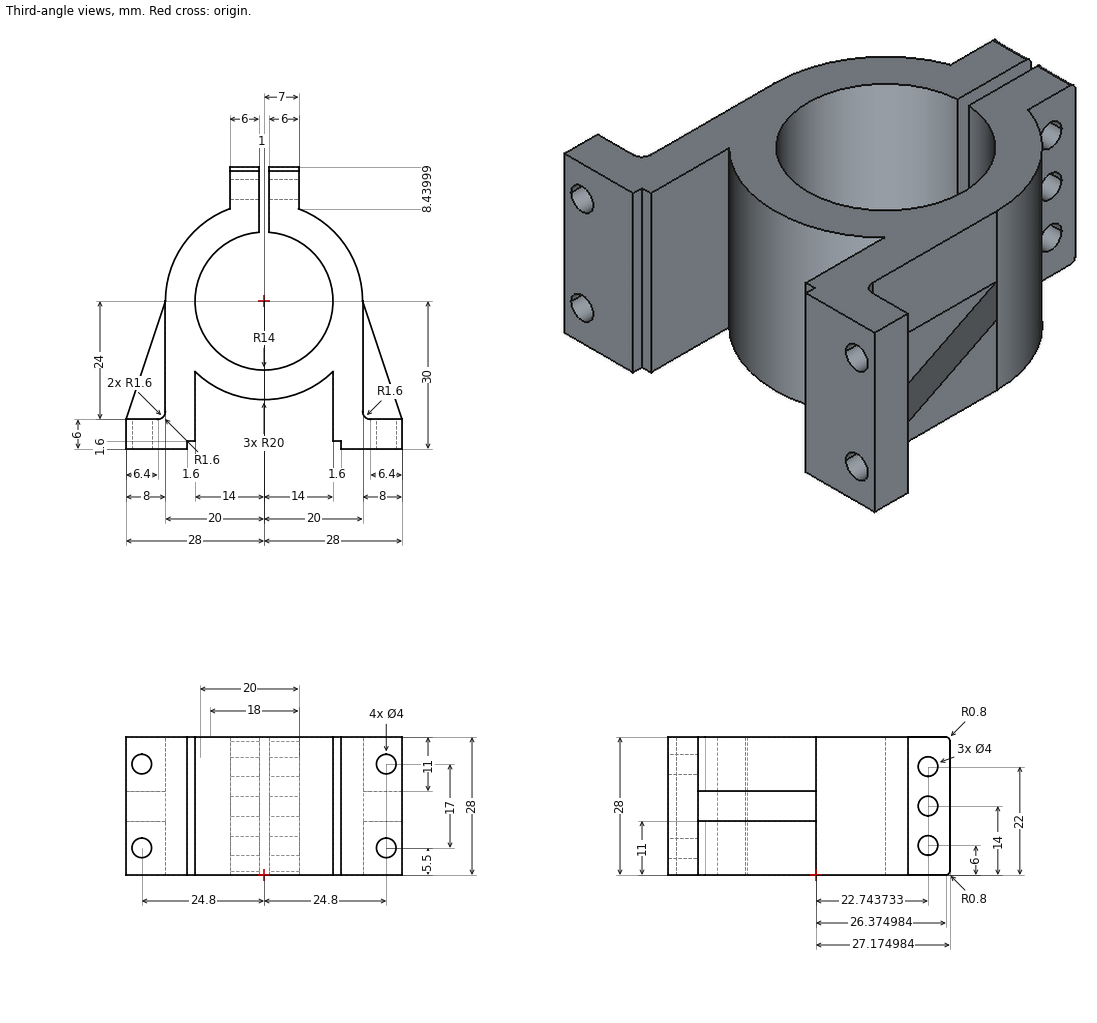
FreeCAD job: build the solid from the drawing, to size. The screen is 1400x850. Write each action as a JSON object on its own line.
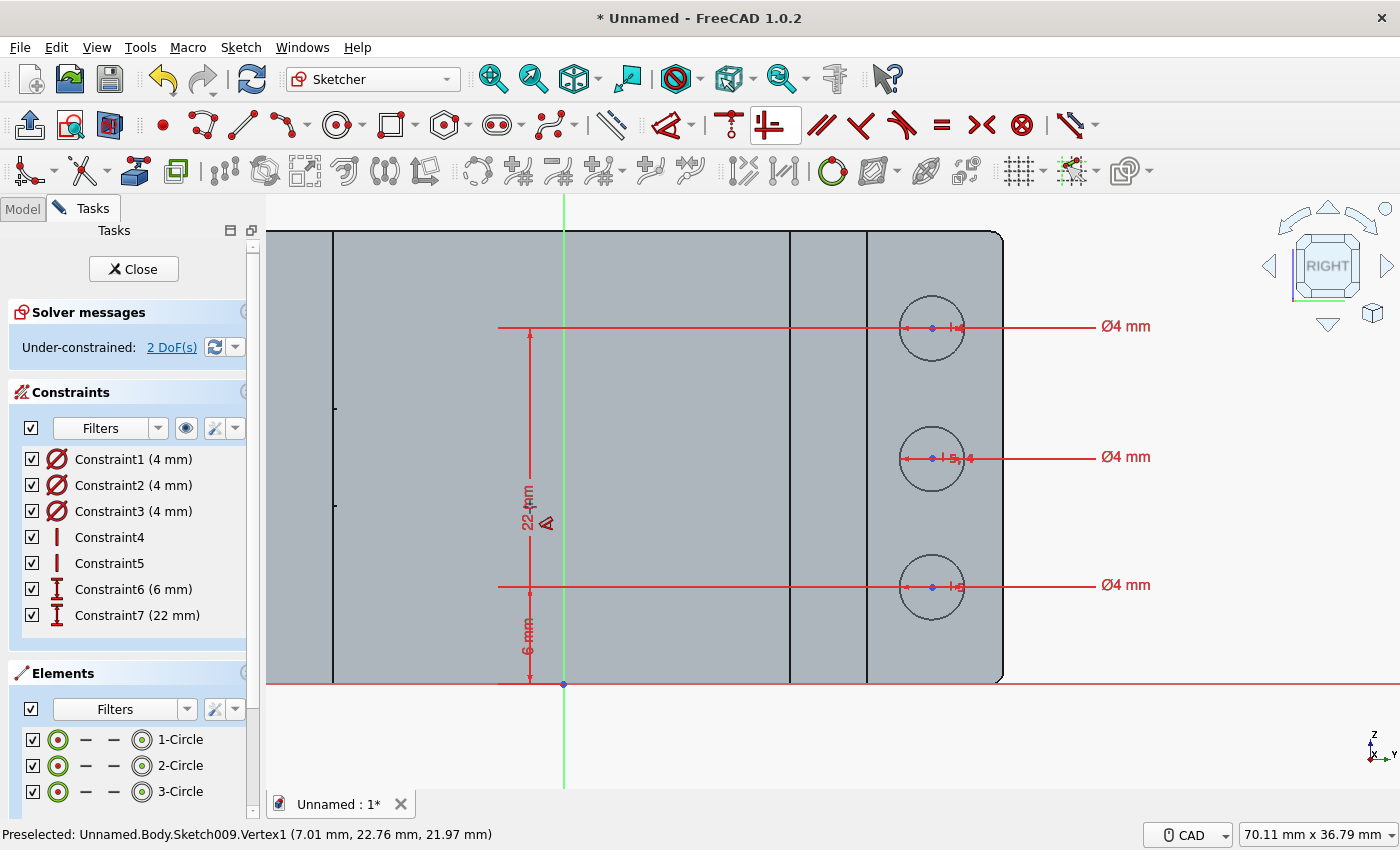
{"action": "left_click", "coordinate": [932, 459]}
{"action": "left_click", "coordinate": [530, 572]}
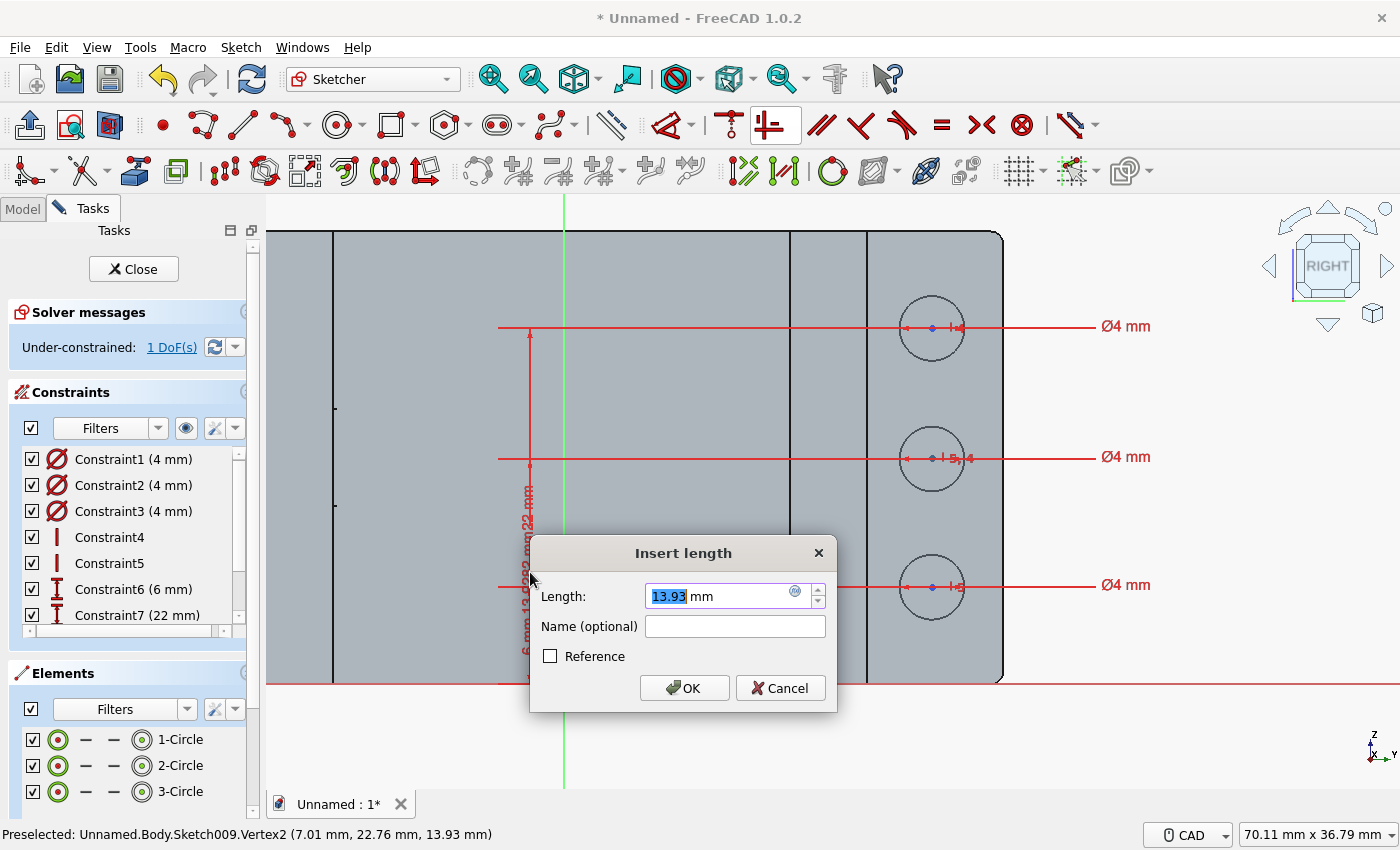
{"action": "type", "text": "14"}
{"action": "key", "text": "Return"}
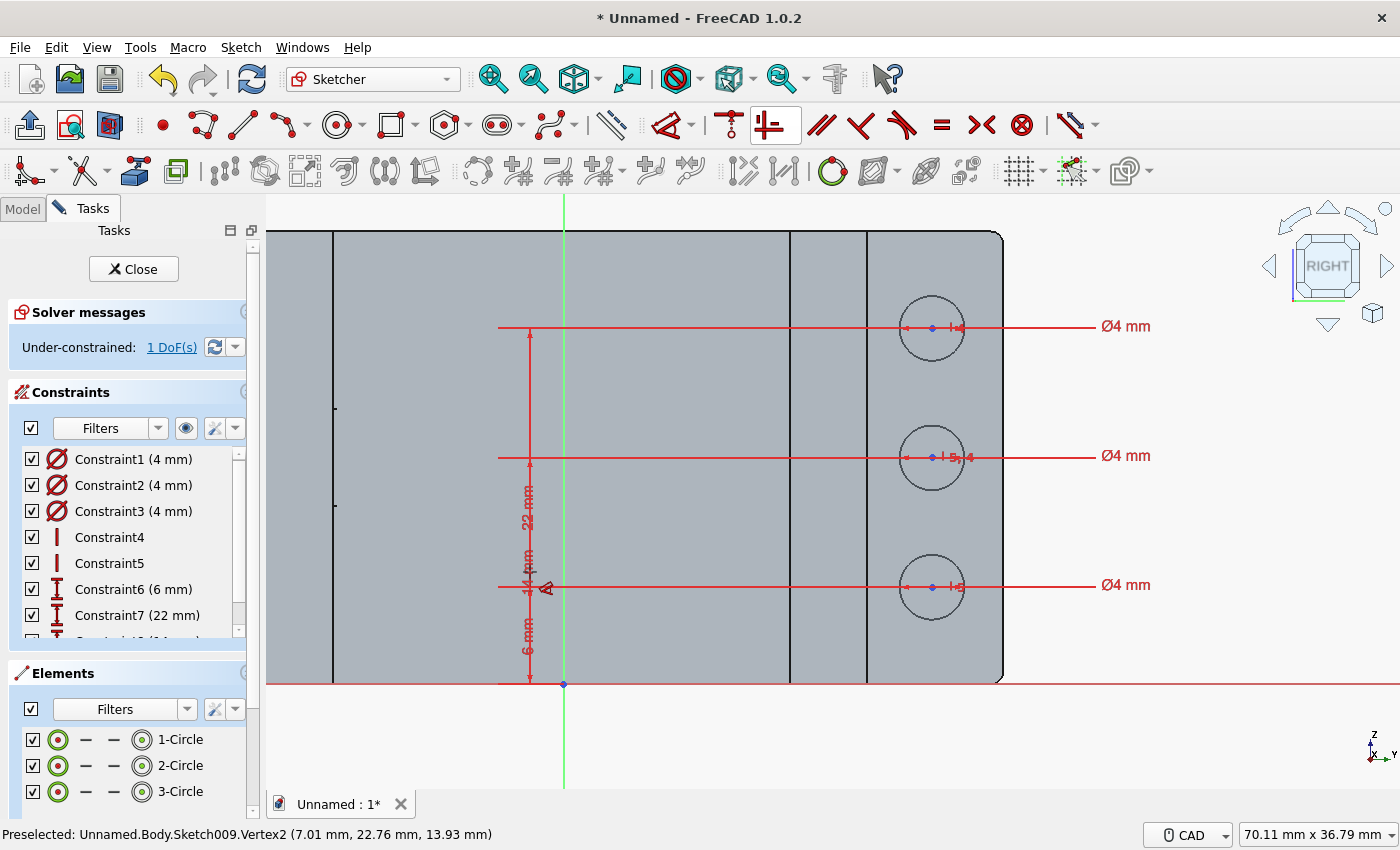
{"action": "left_click", "coordinate": [932, 328]}
{"action": "left_click", "coordinate": [748, 718]}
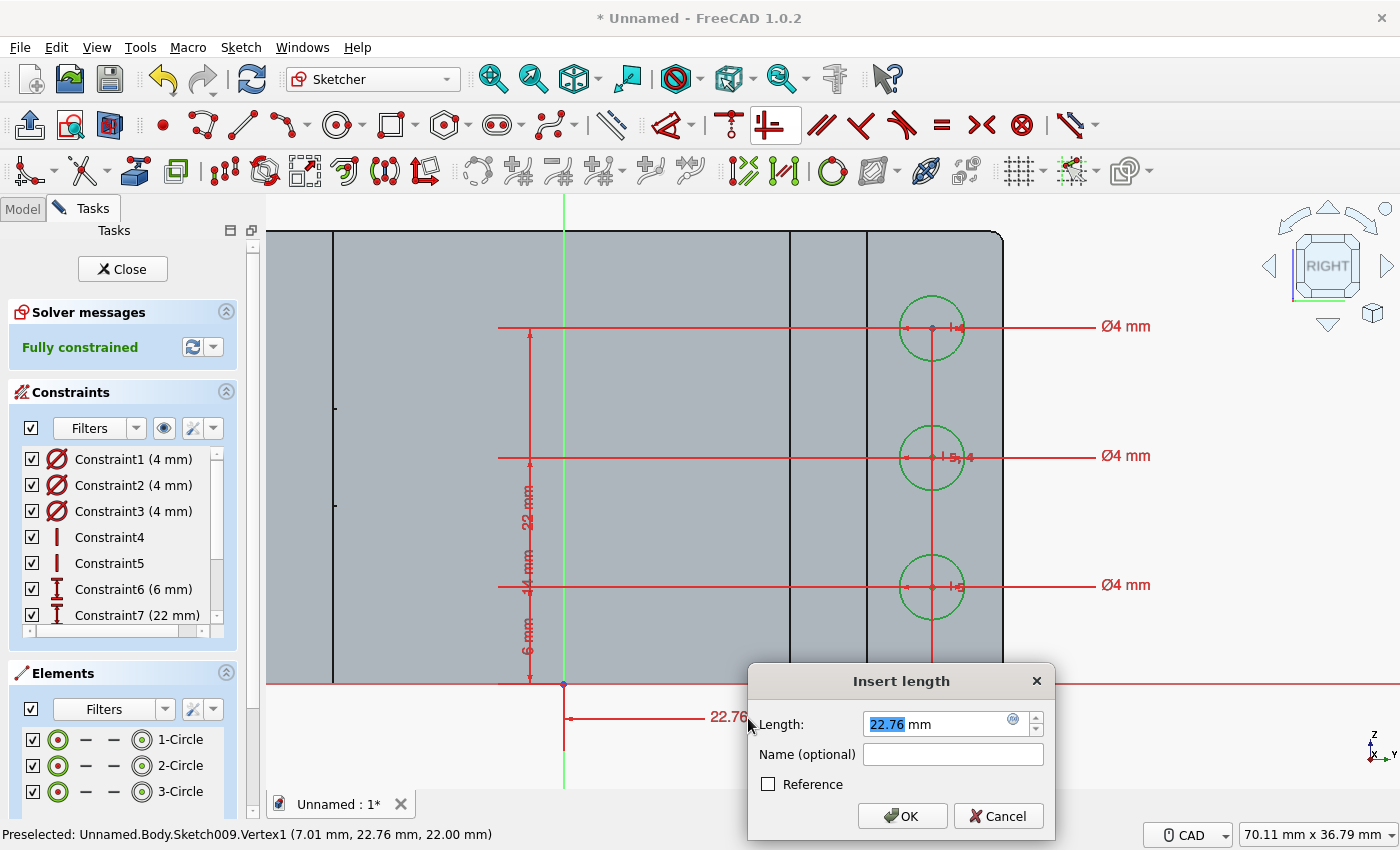
{"action": "type", "text": "22.743733"}
{"action": "key", "text": "Return"}
{"action": "key", "text": "Escape"}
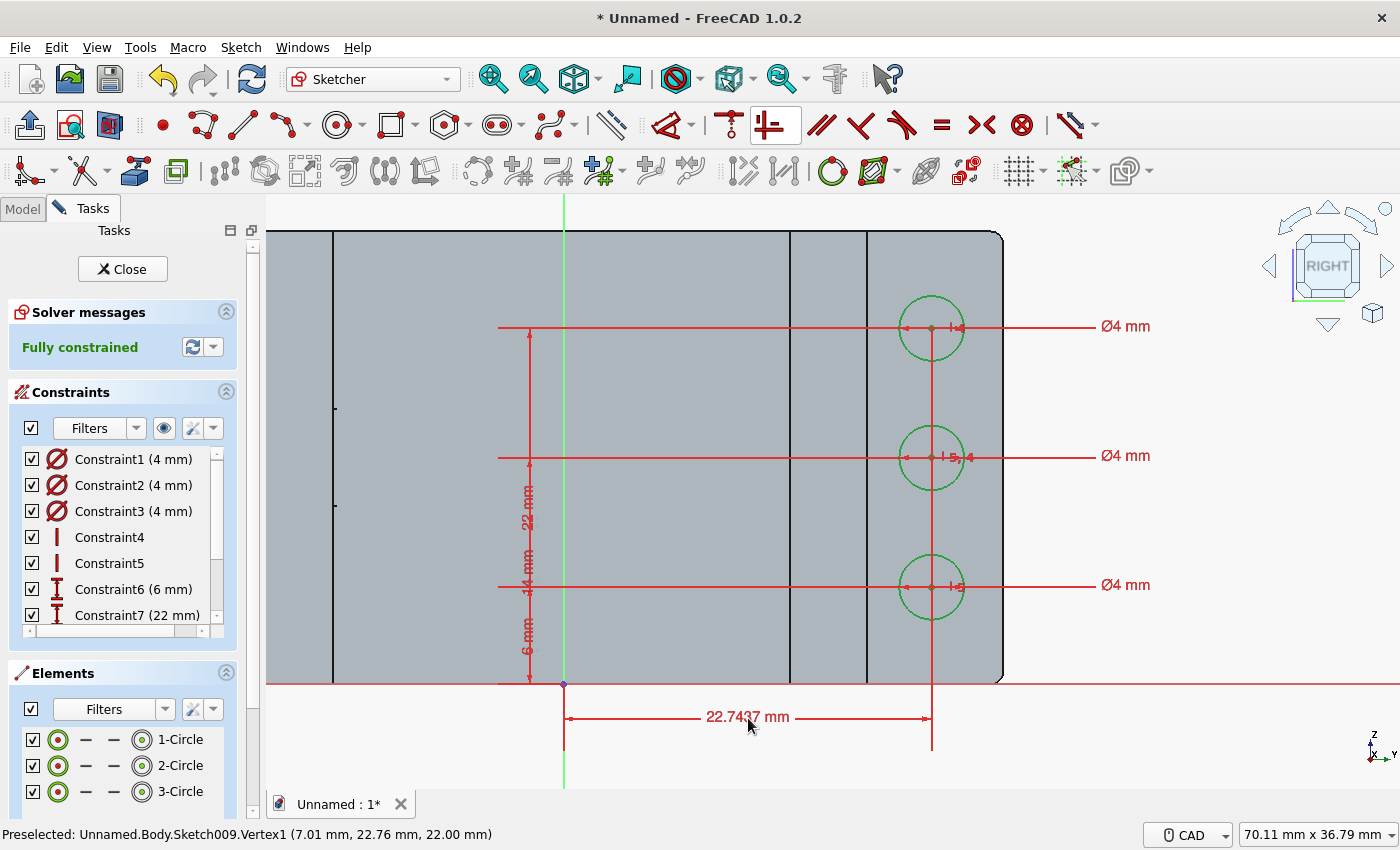
{"action": "left_click", "coordinate": [123, 269]}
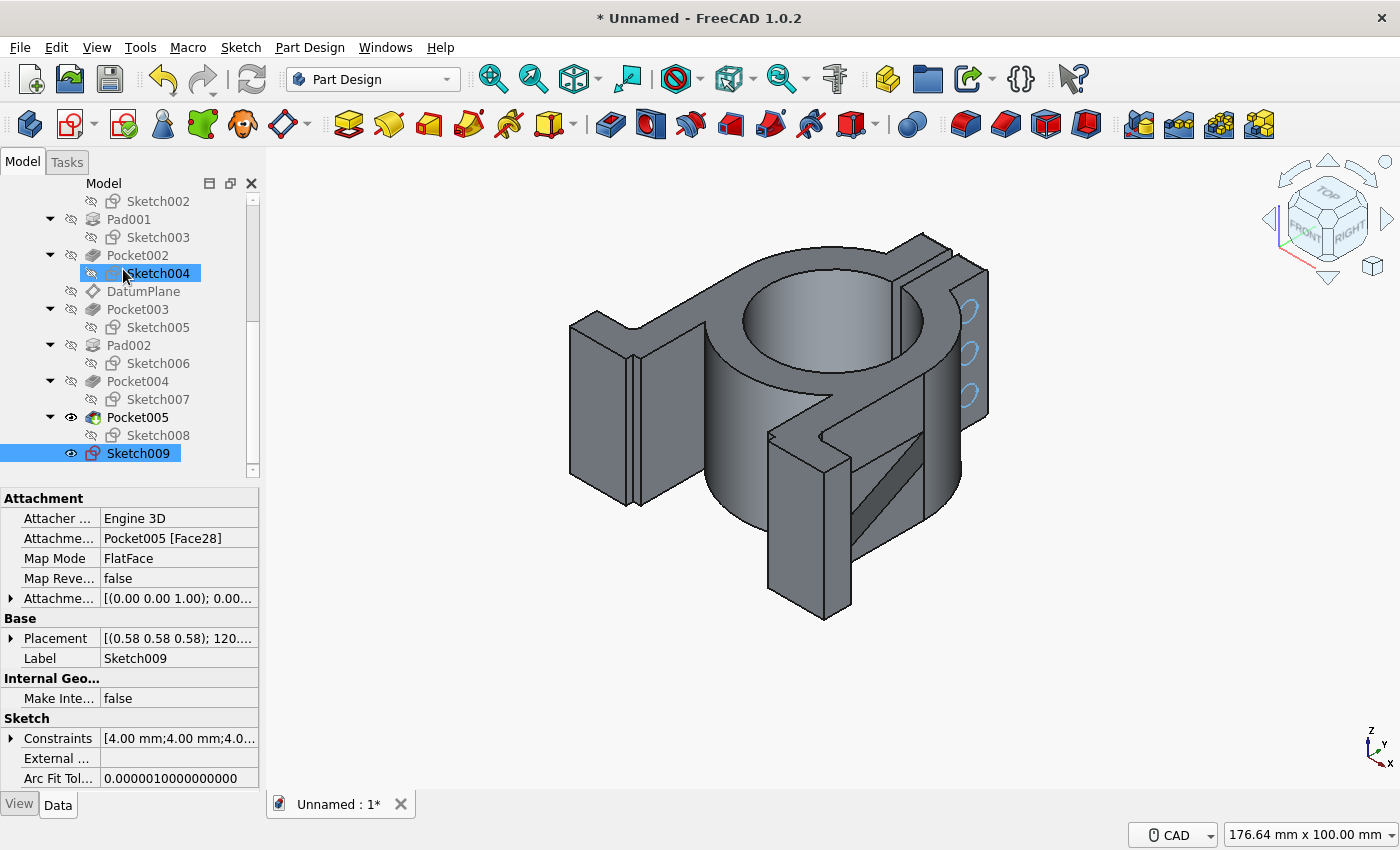
{"action": "left_click", "coordinate": [612, 124]}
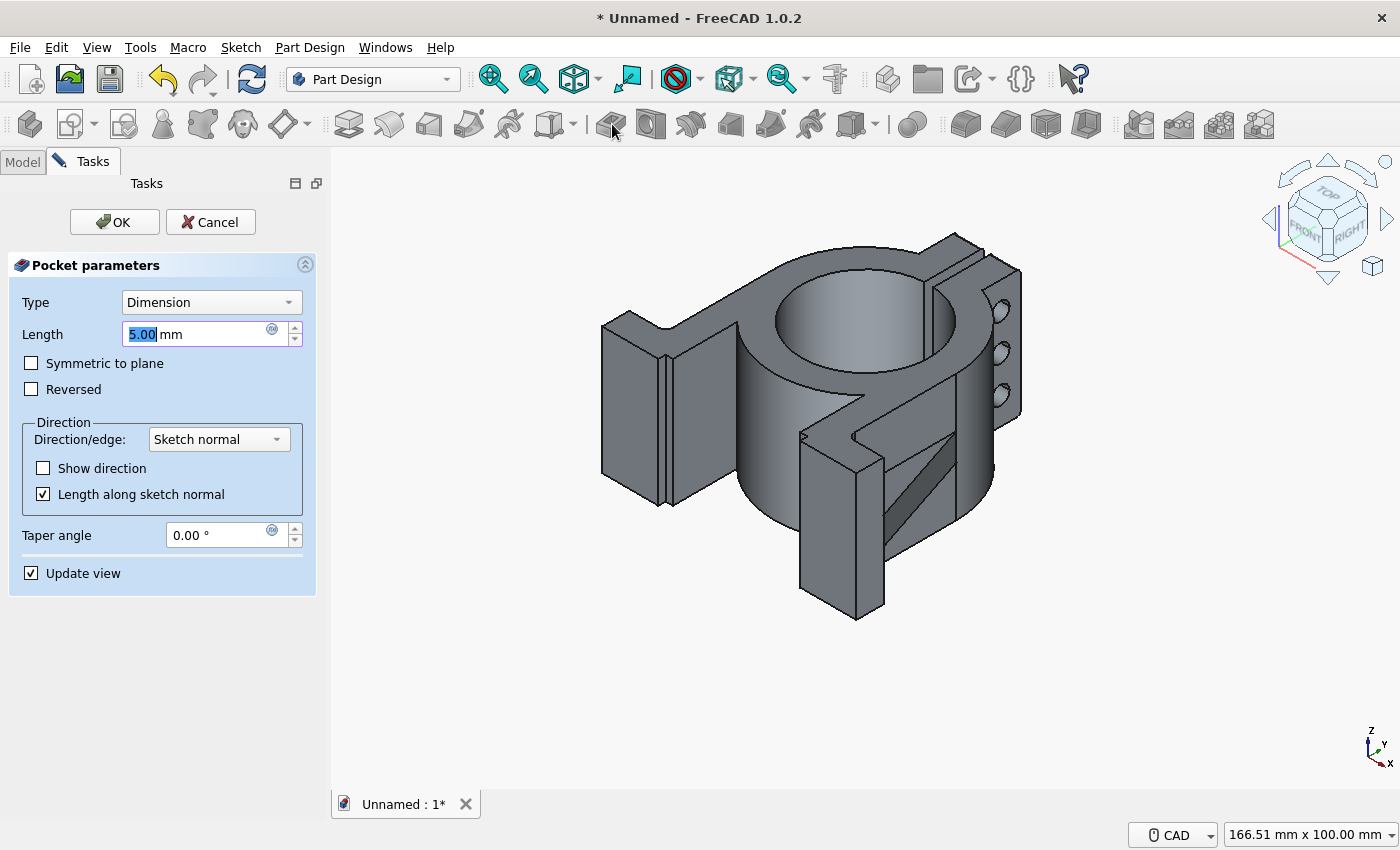
{"action": "type", "text": "20"}
{"action": "key", "text": "Tab"}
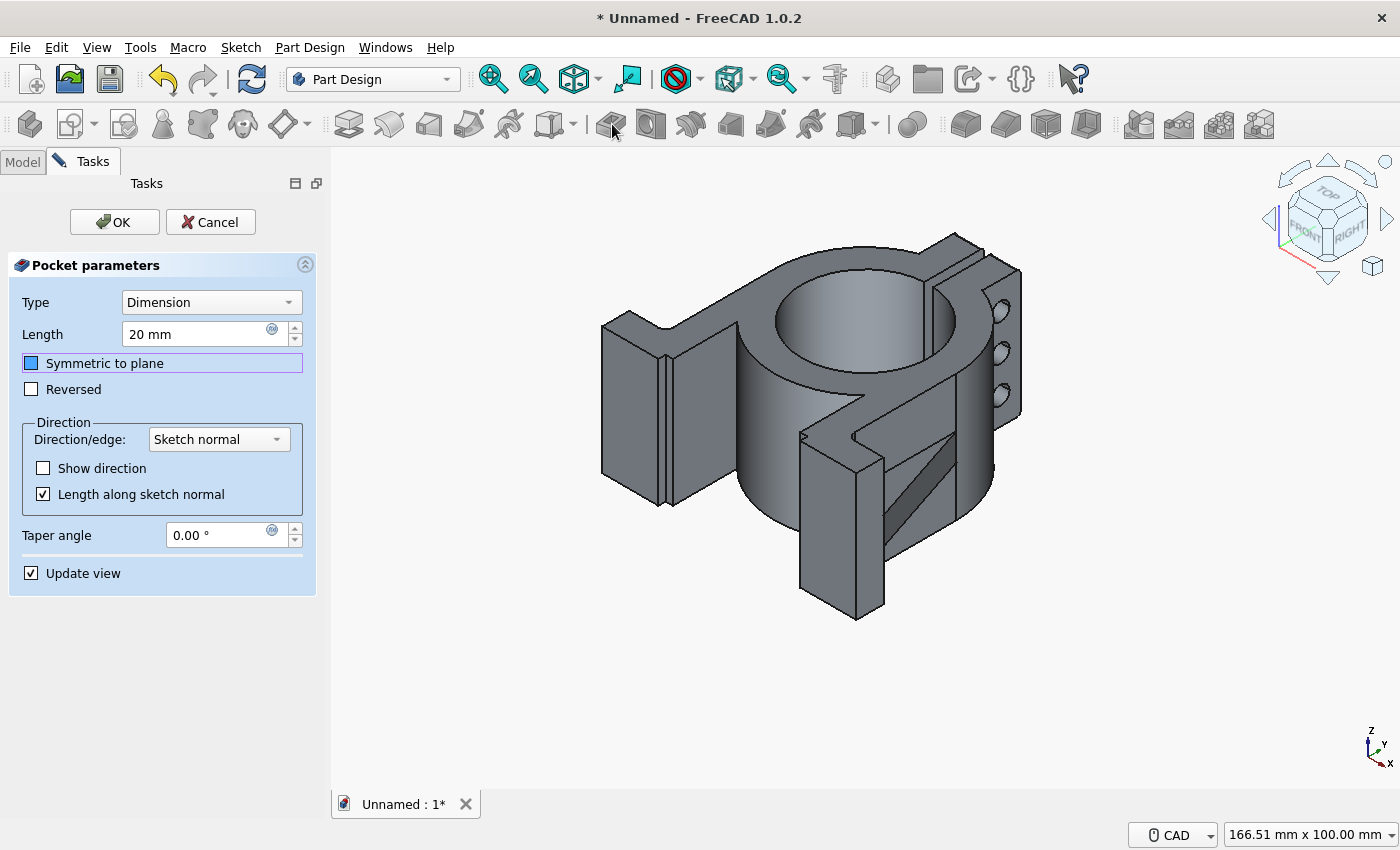
{"action": "left_click", "coordinate": [115, 222]}